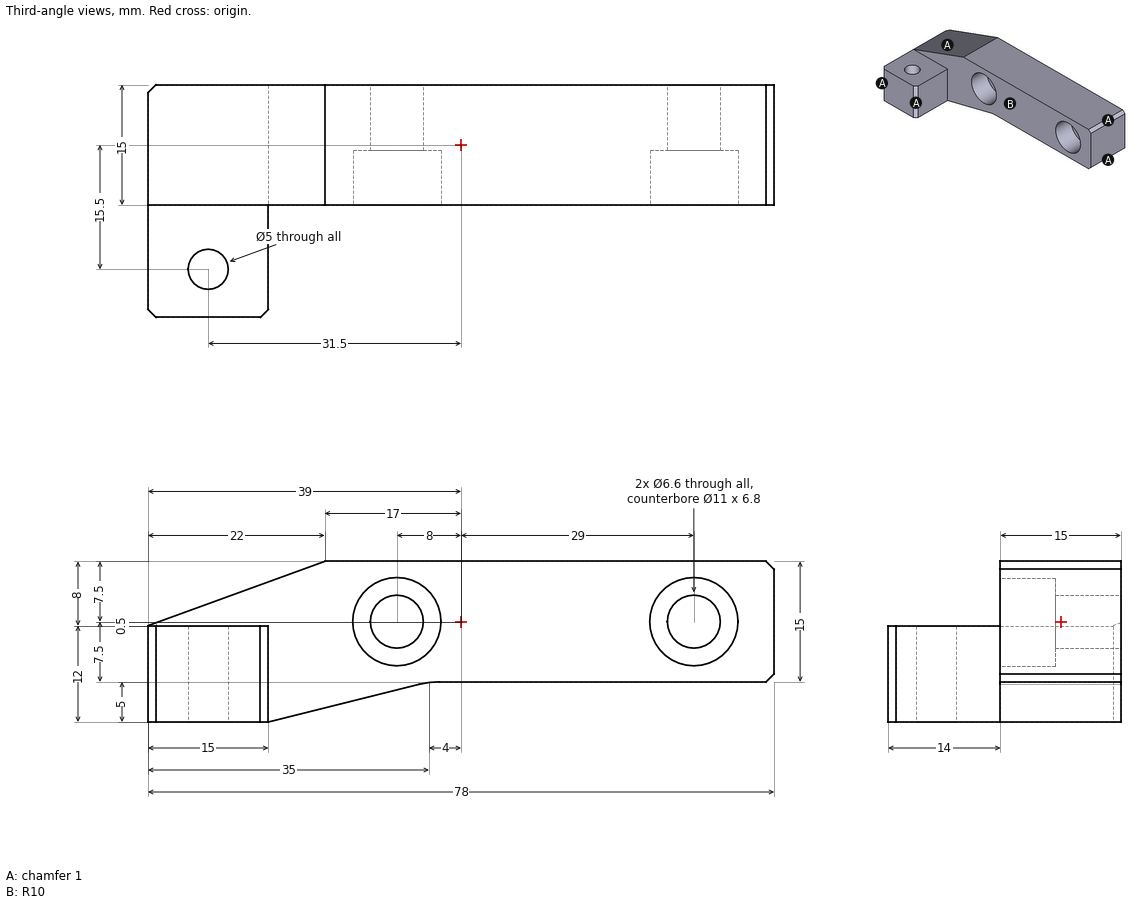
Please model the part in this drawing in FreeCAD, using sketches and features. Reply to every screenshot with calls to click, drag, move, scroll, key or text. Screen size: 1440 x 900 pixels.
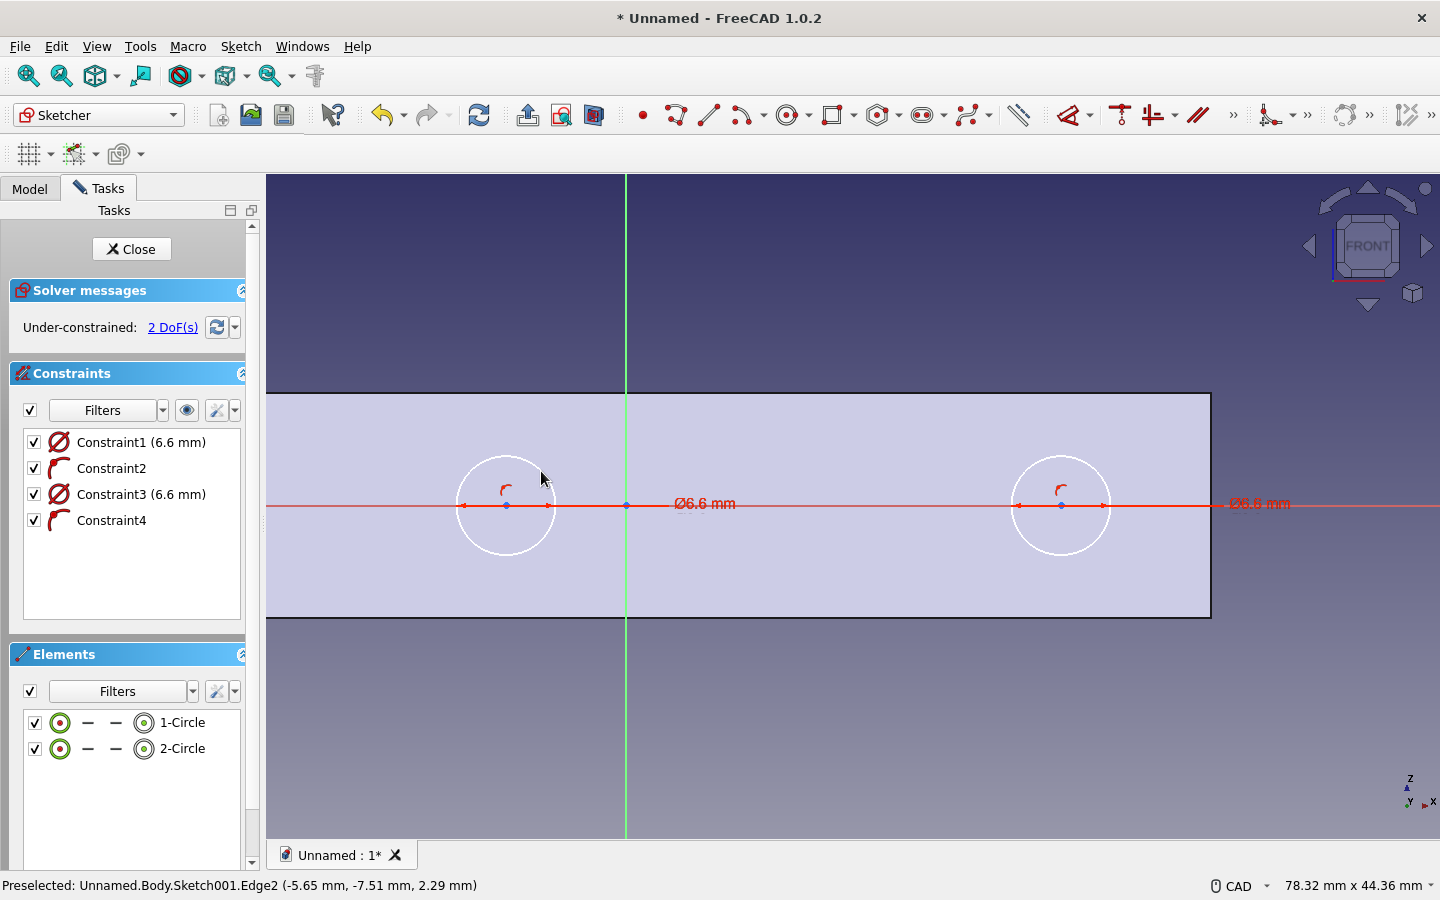
click(506, 506)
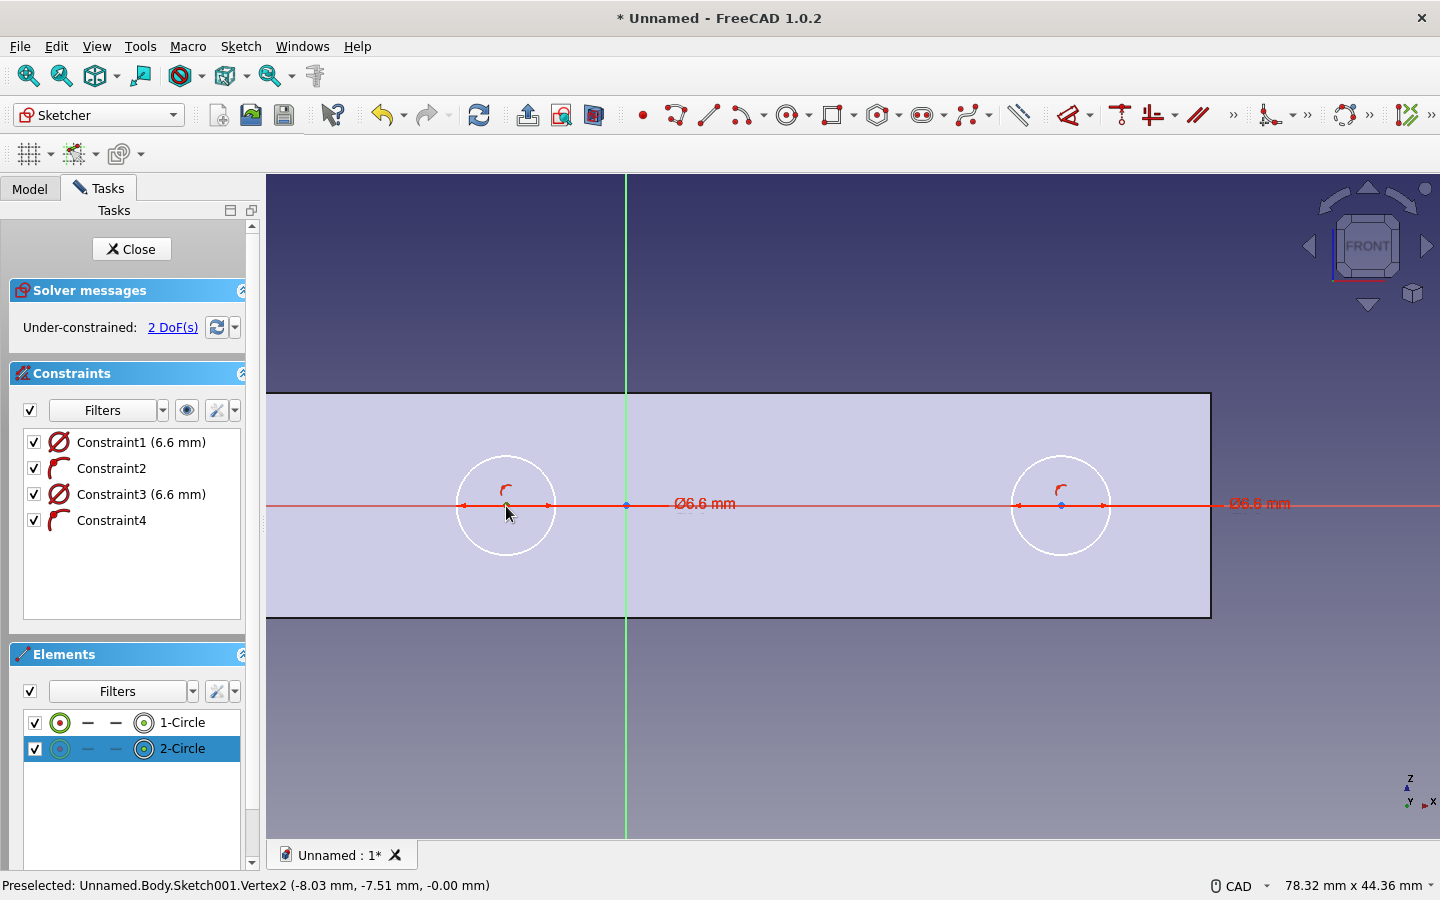
key(l)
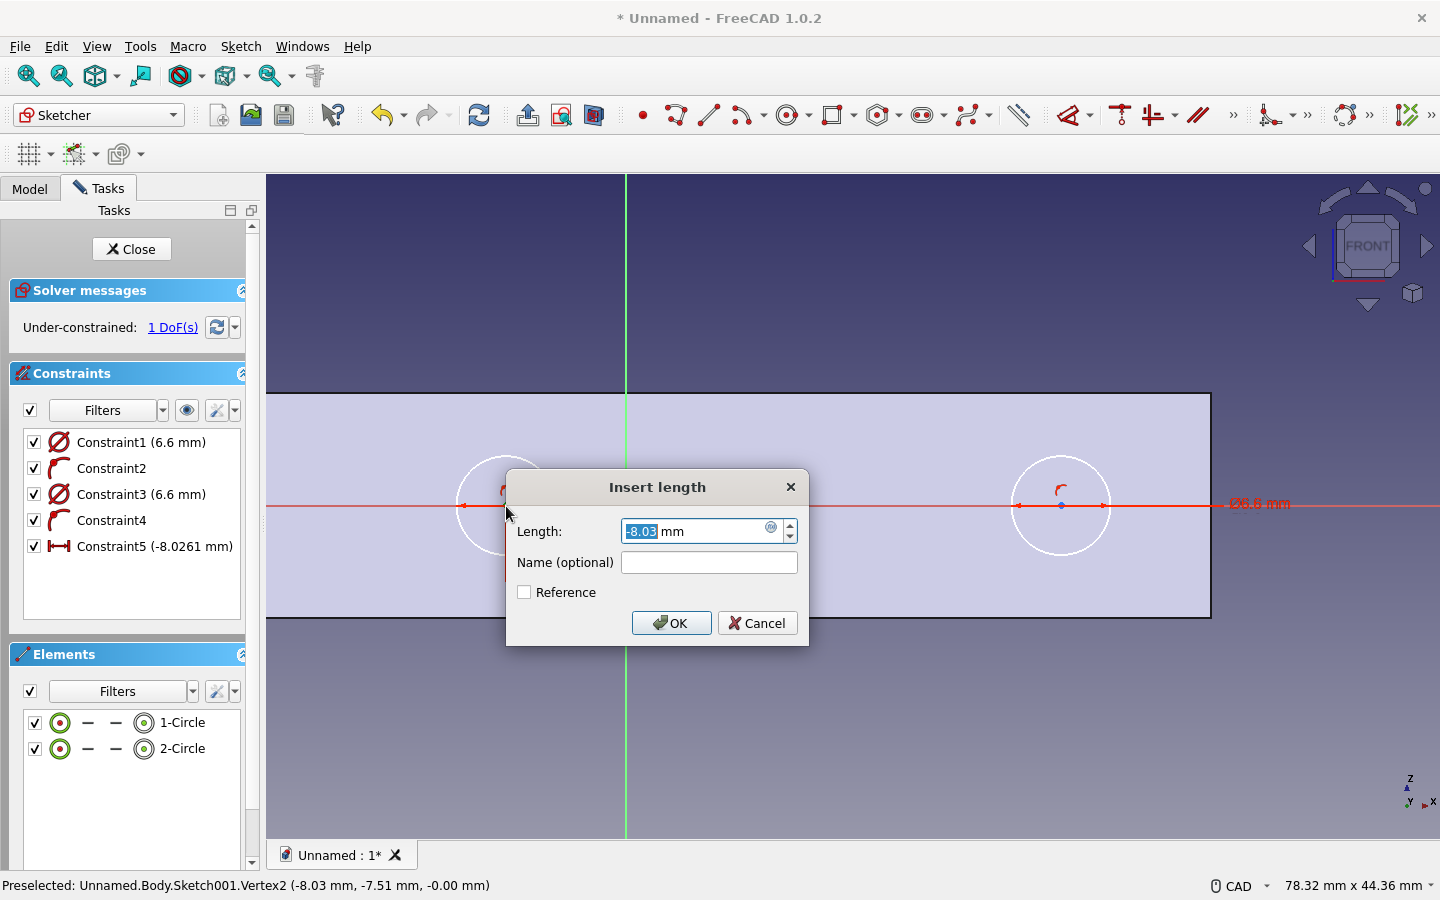
text(-8)
key(Return)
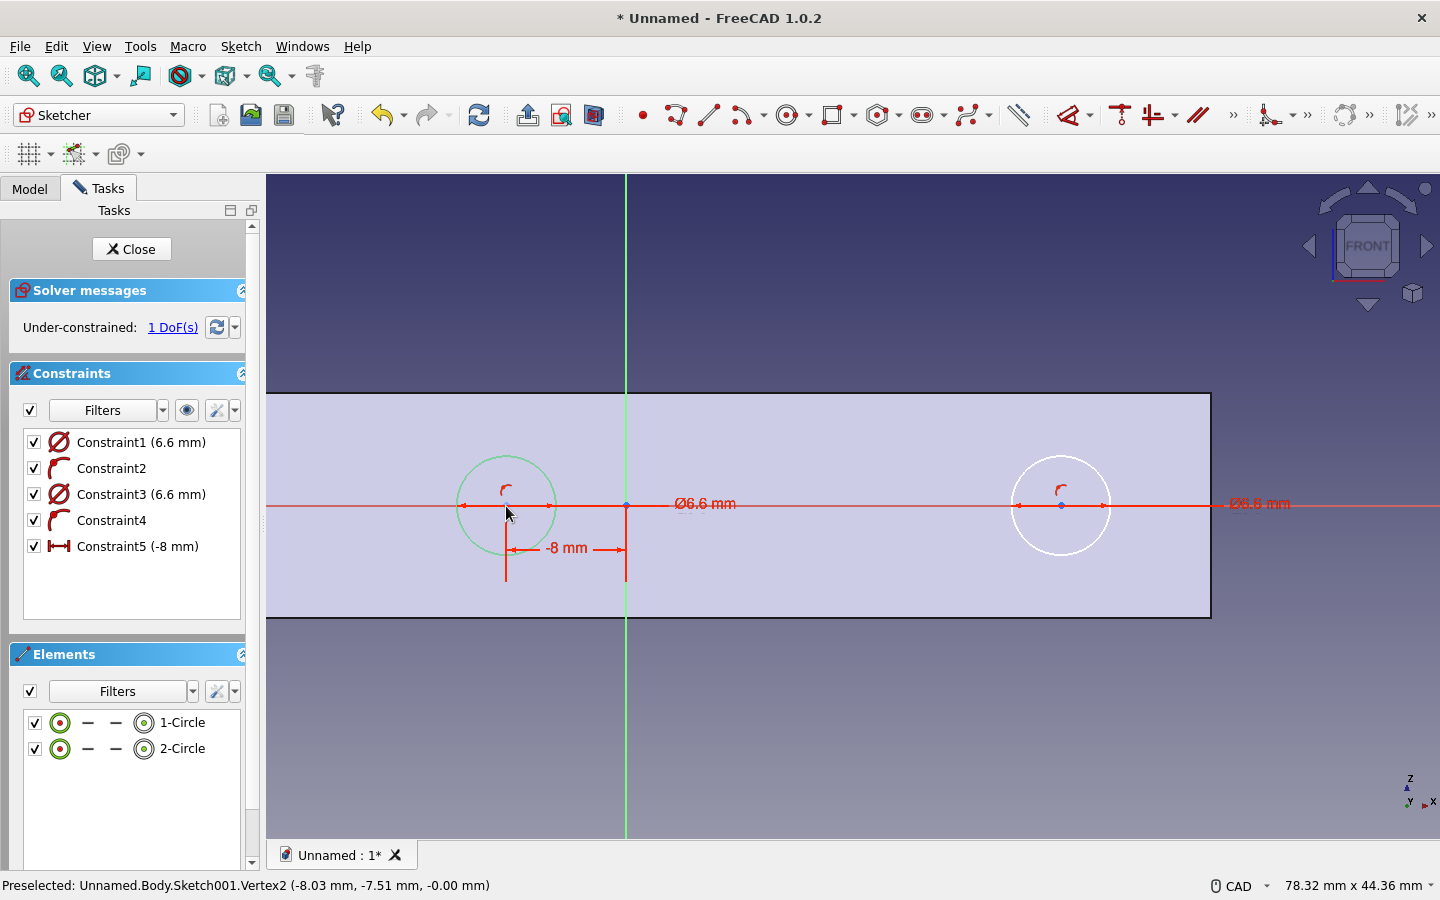
click(1061, 506)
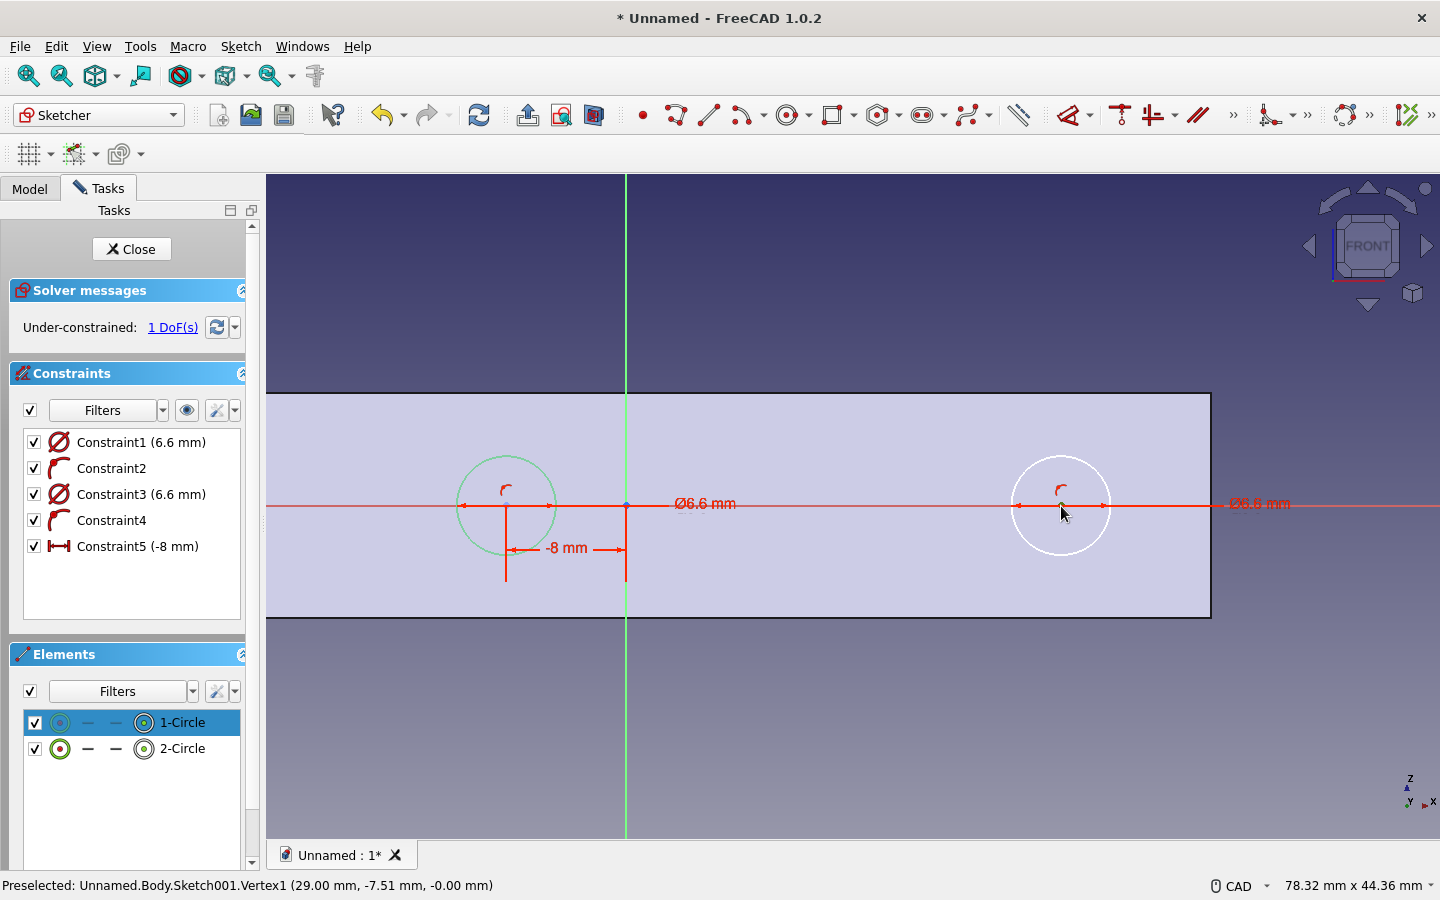
key(l)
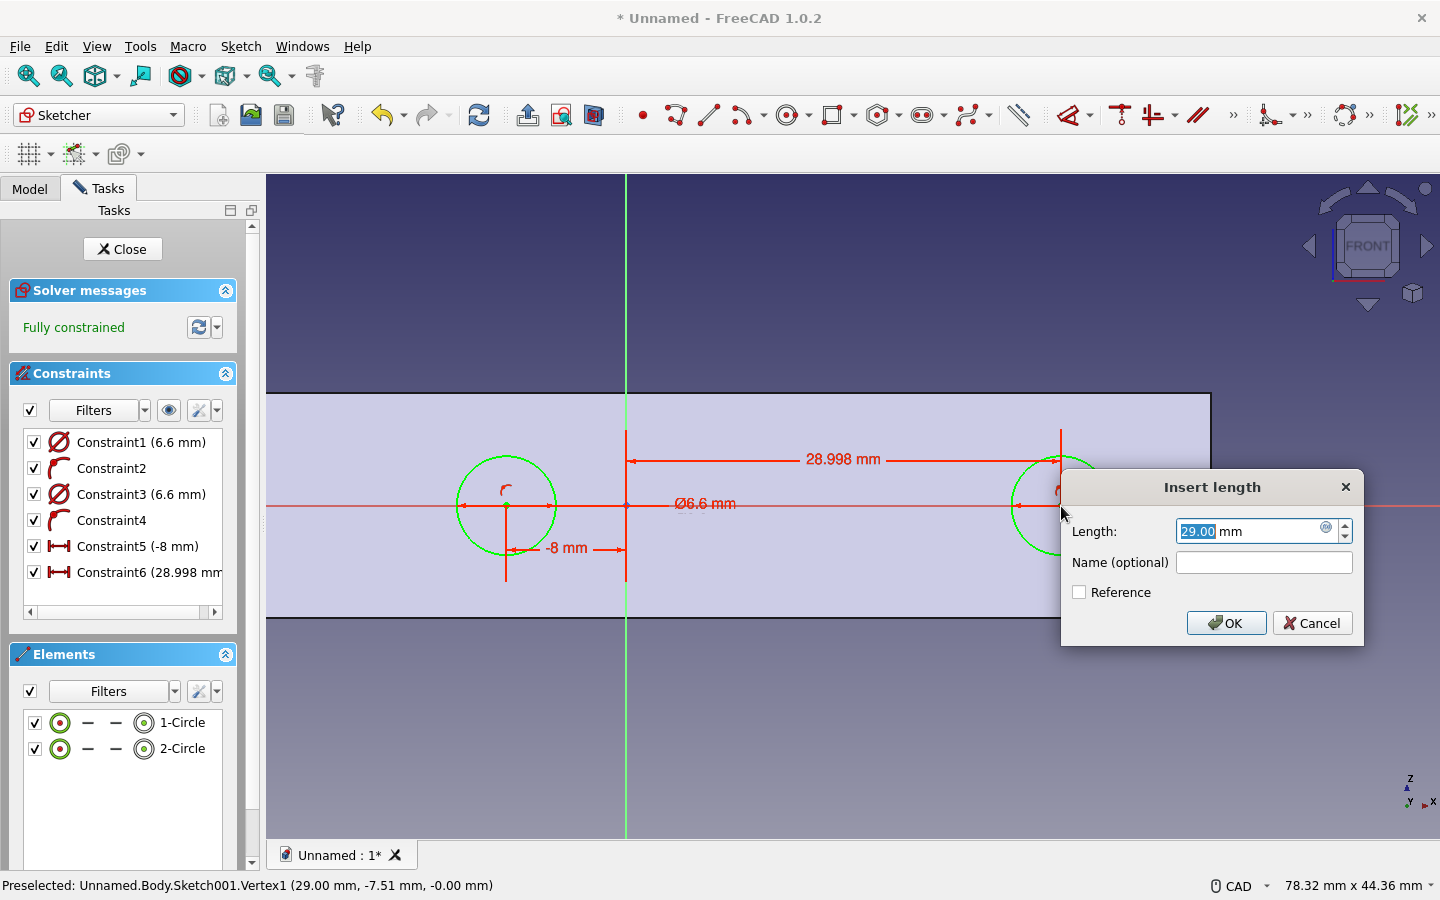
text(29)
key(Return)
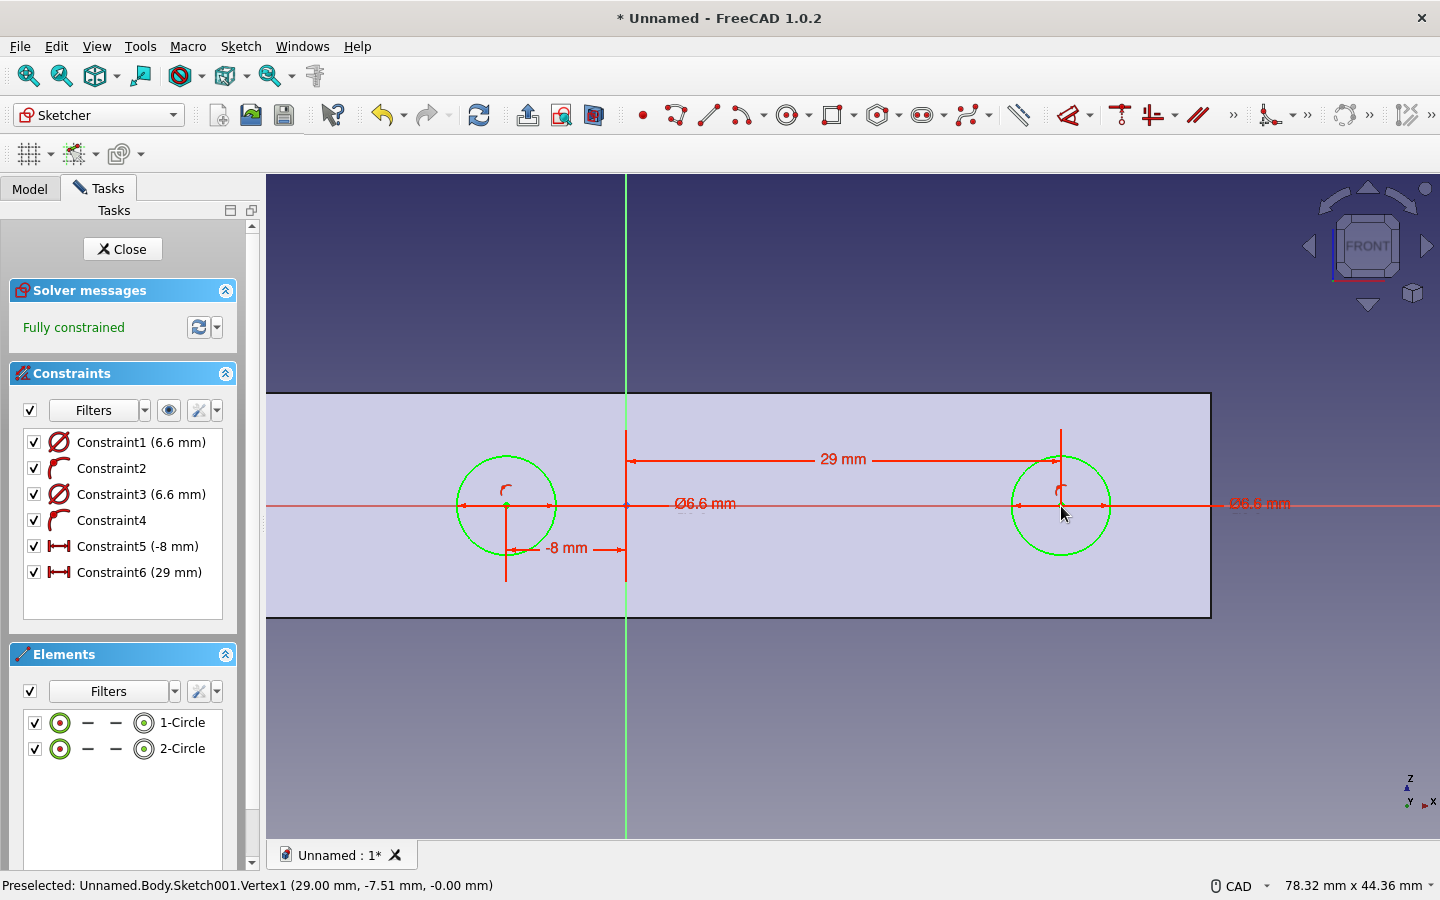
click(123, 249)